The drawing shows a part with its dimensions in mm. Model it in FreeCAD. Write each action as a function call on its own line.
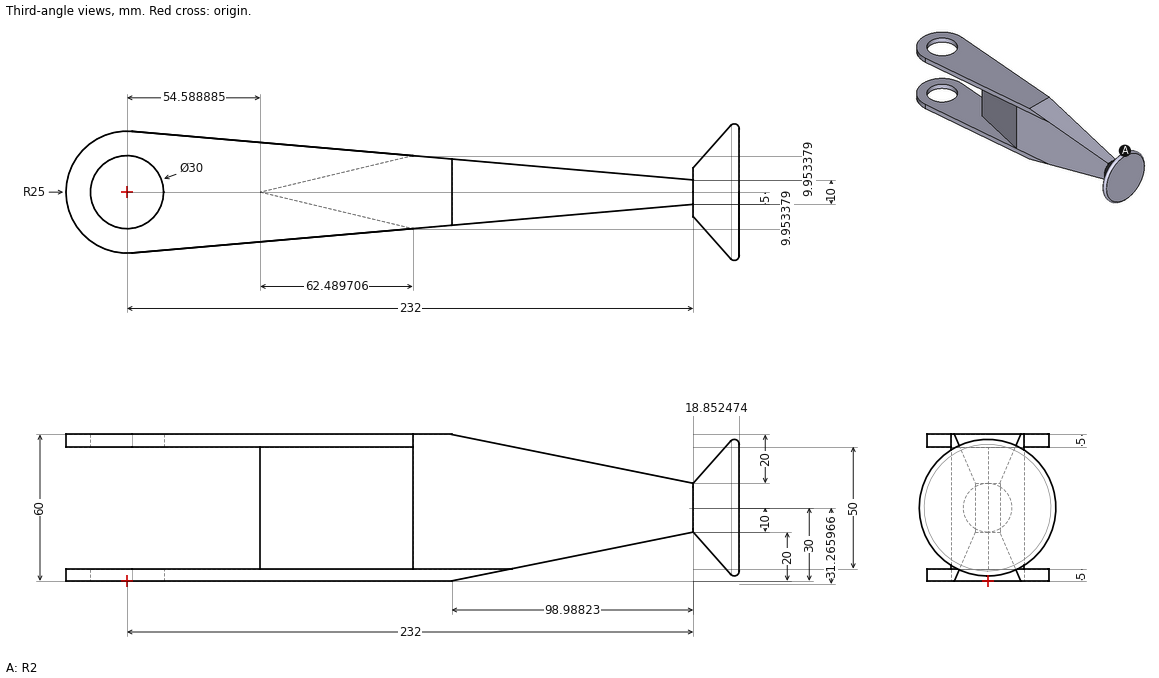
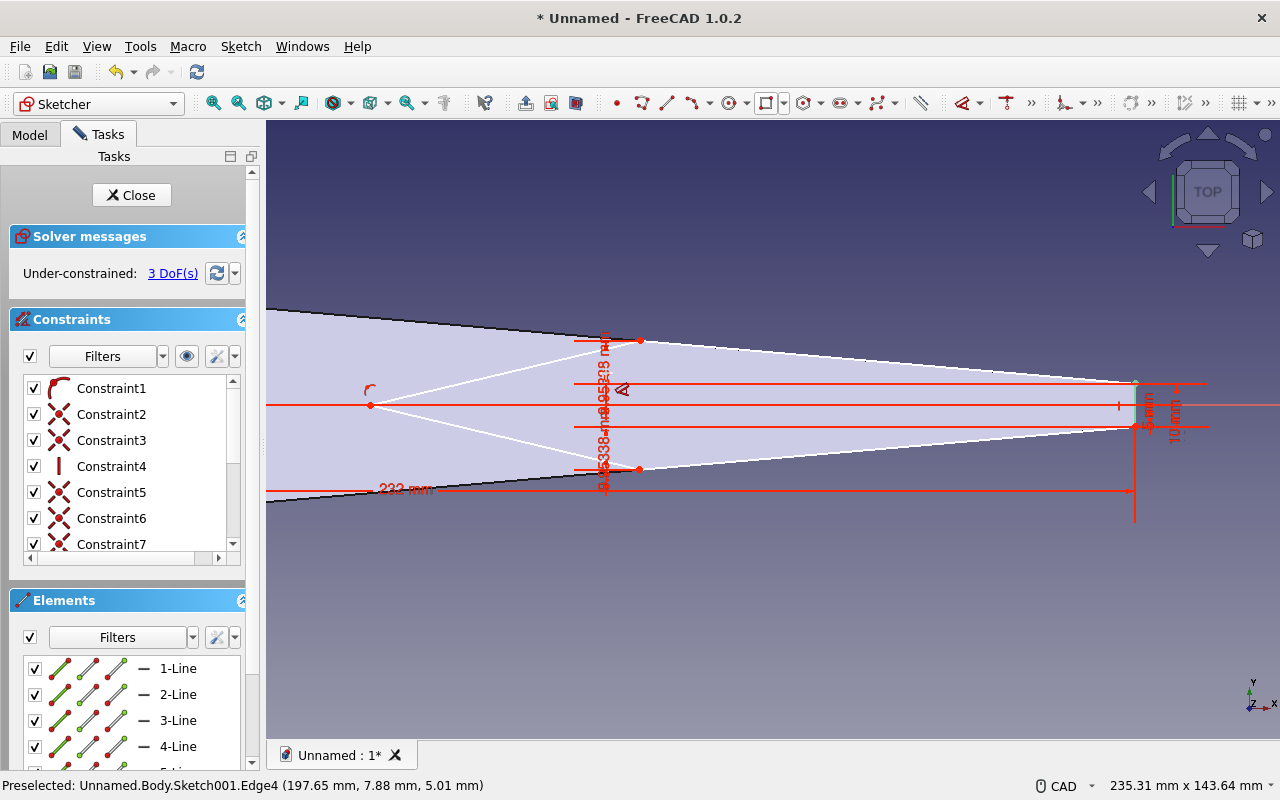
click(370, 405)
click(332, 439)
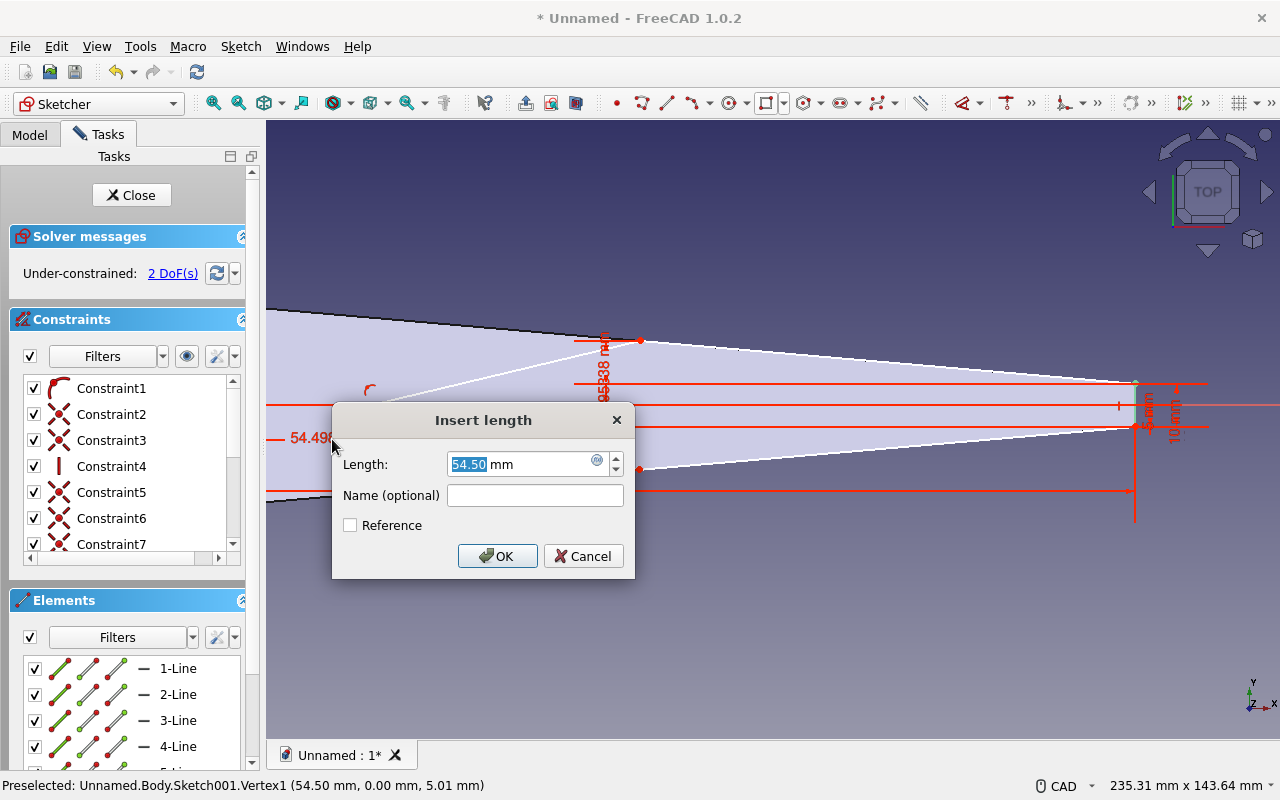
text(54.588885)
key(Return)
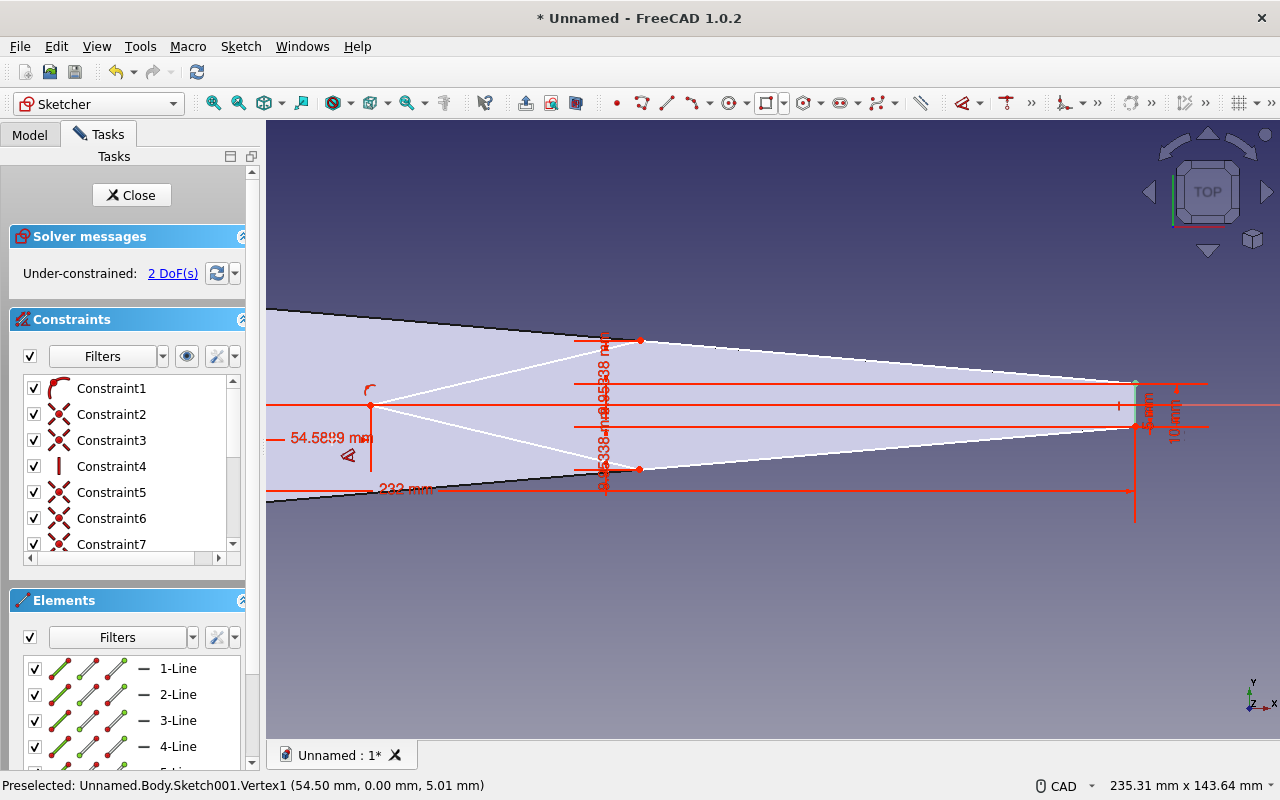
click(451, 425)
click(505, 504)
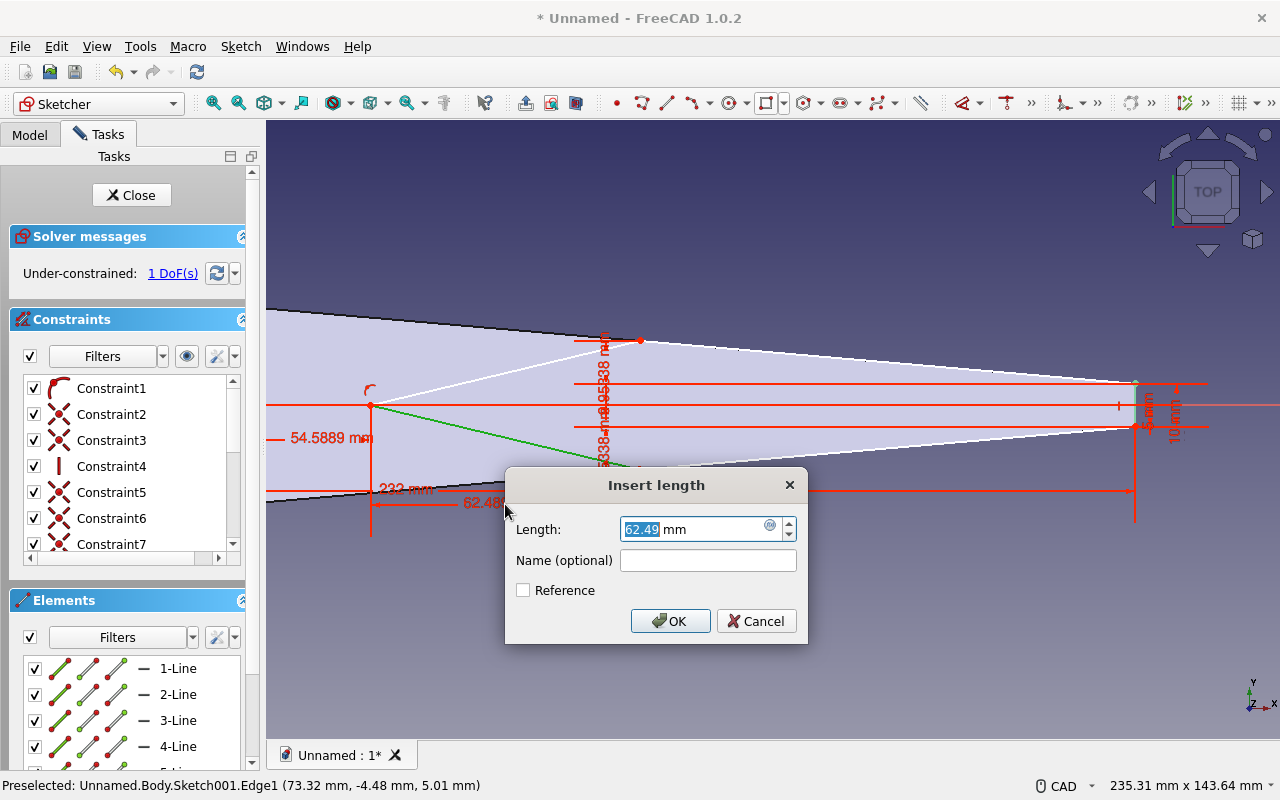
text(62.489706)
key(Return)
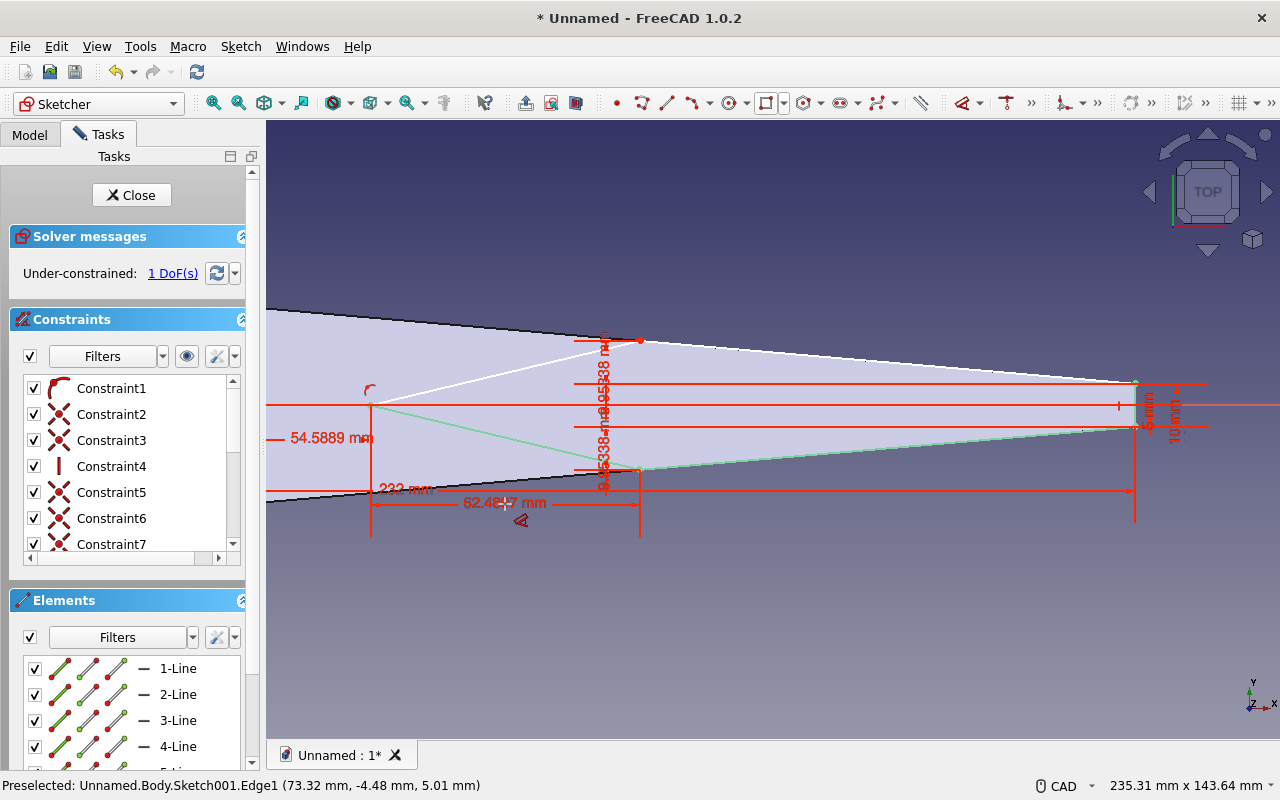
click(559, 360)
click(505, 307)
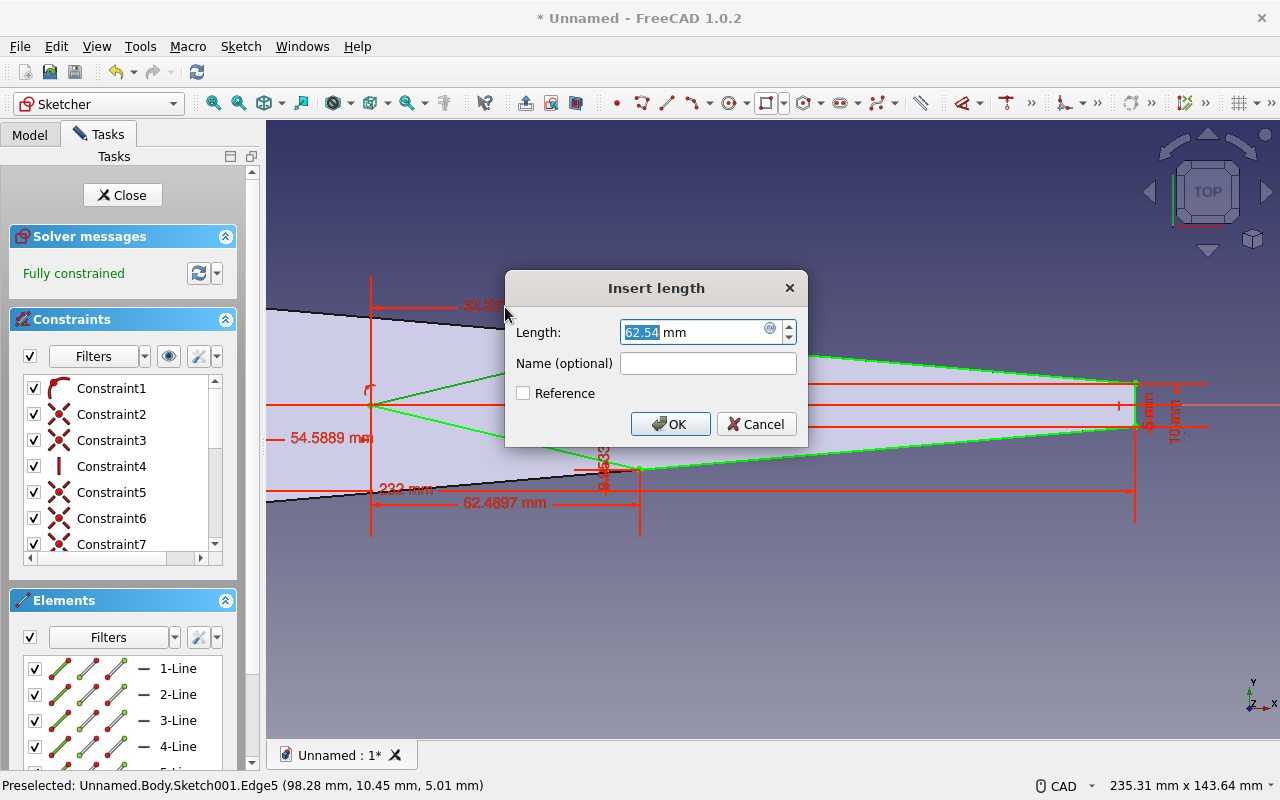
text(62.489706)
key(Return)
key(Escape)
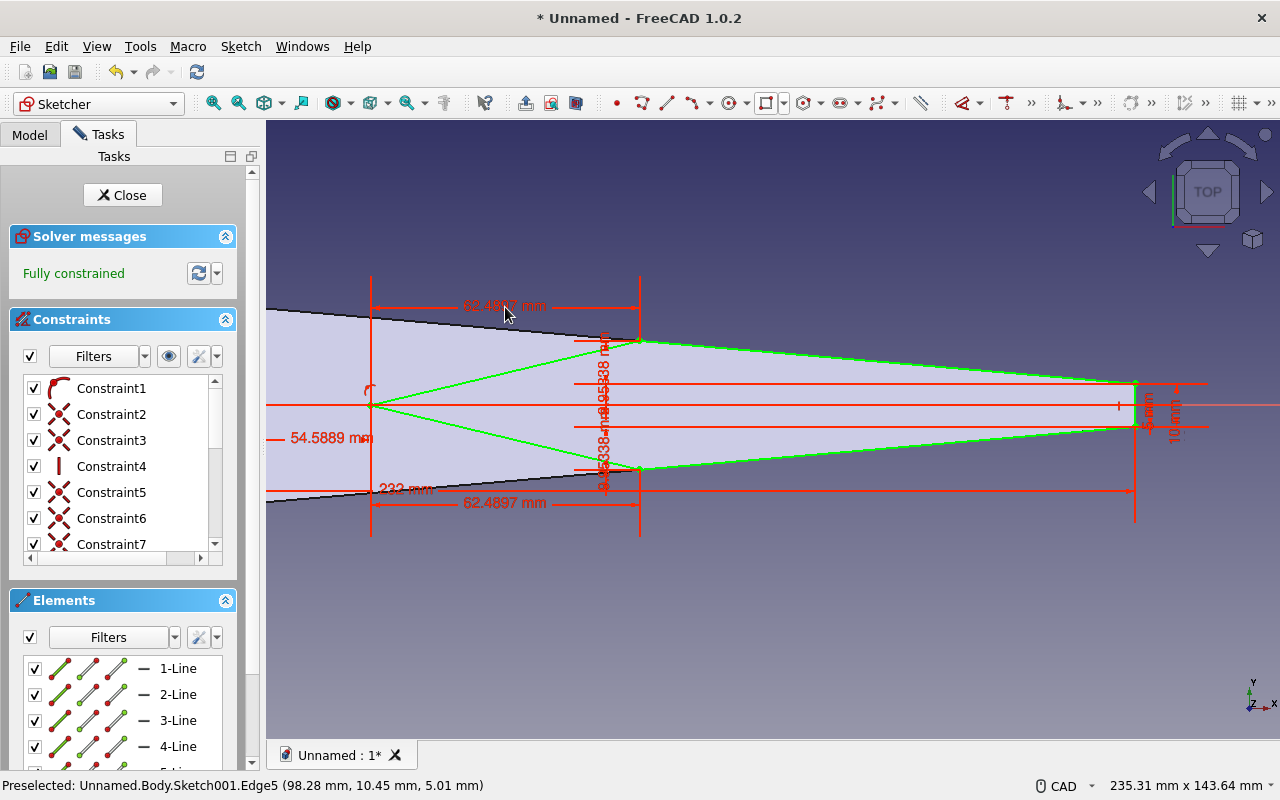
click(123, 195)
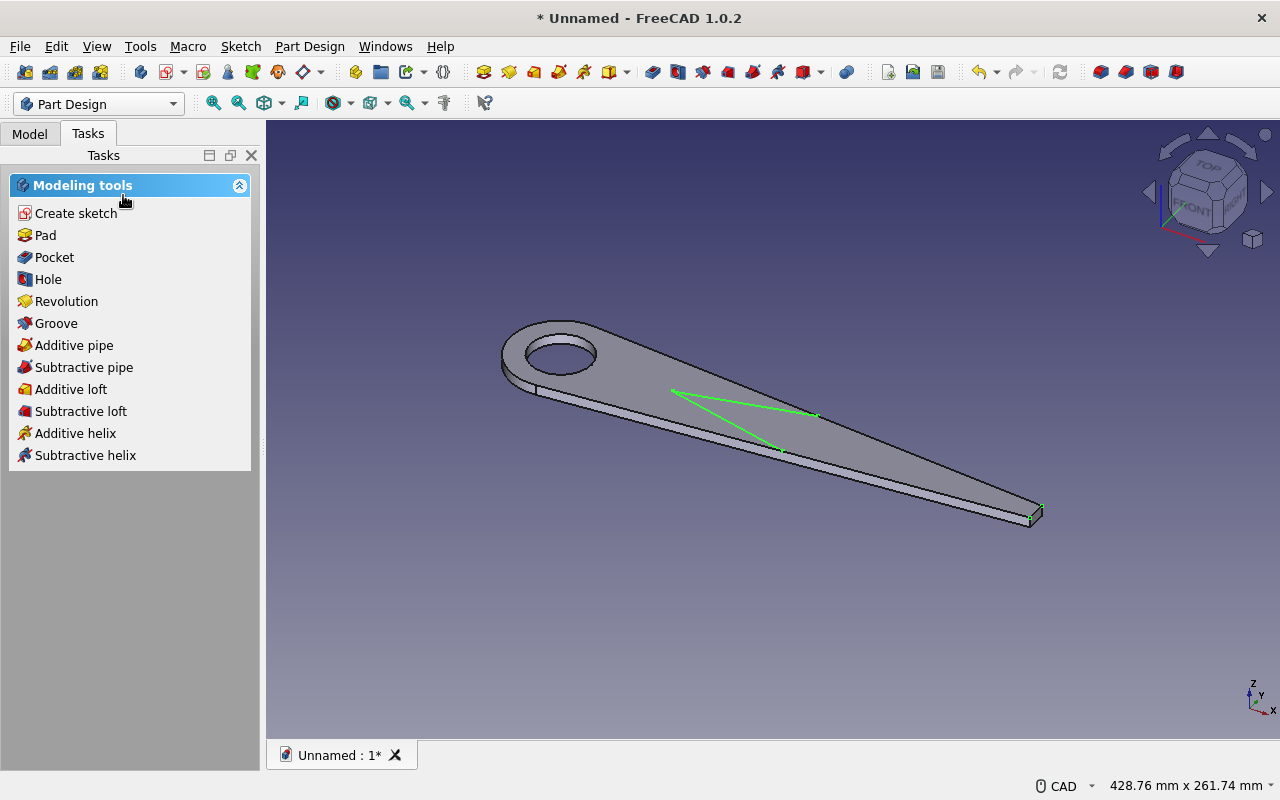
click(484, 72)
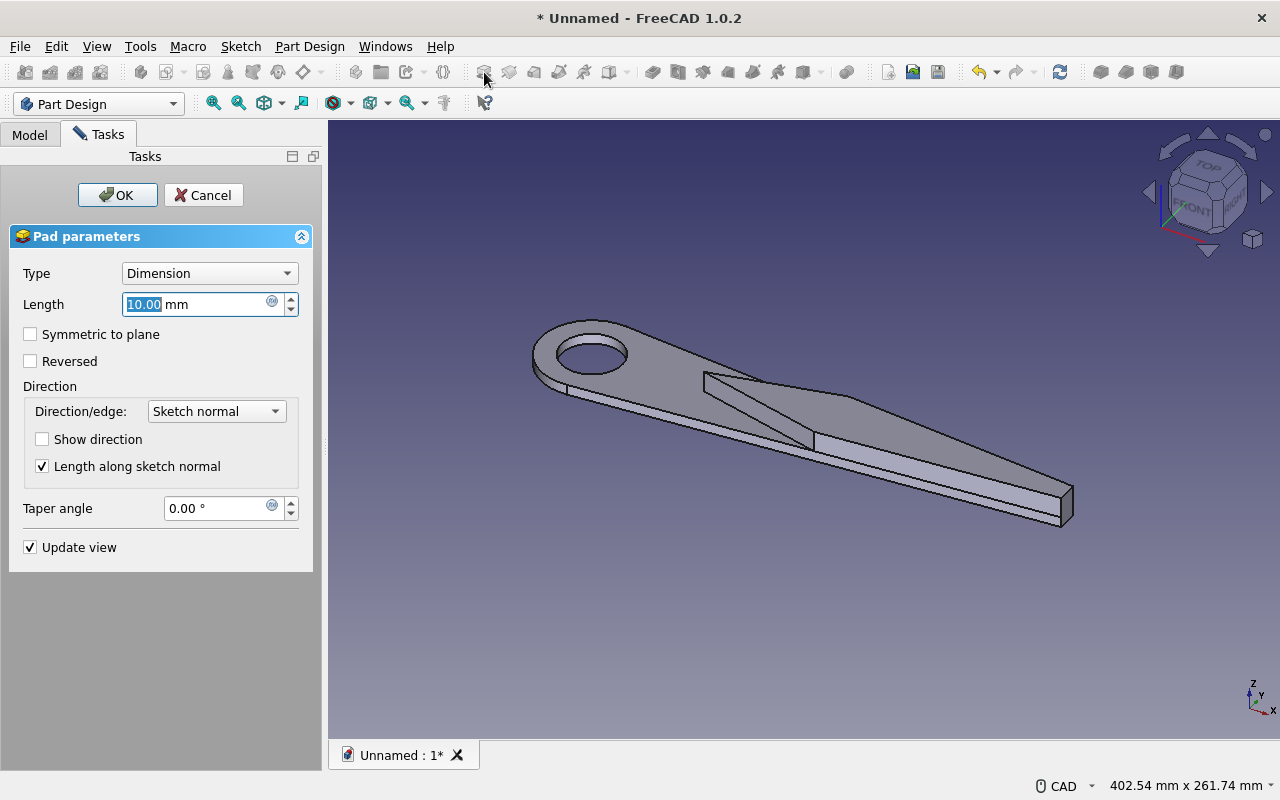
text(50)
key(Tab)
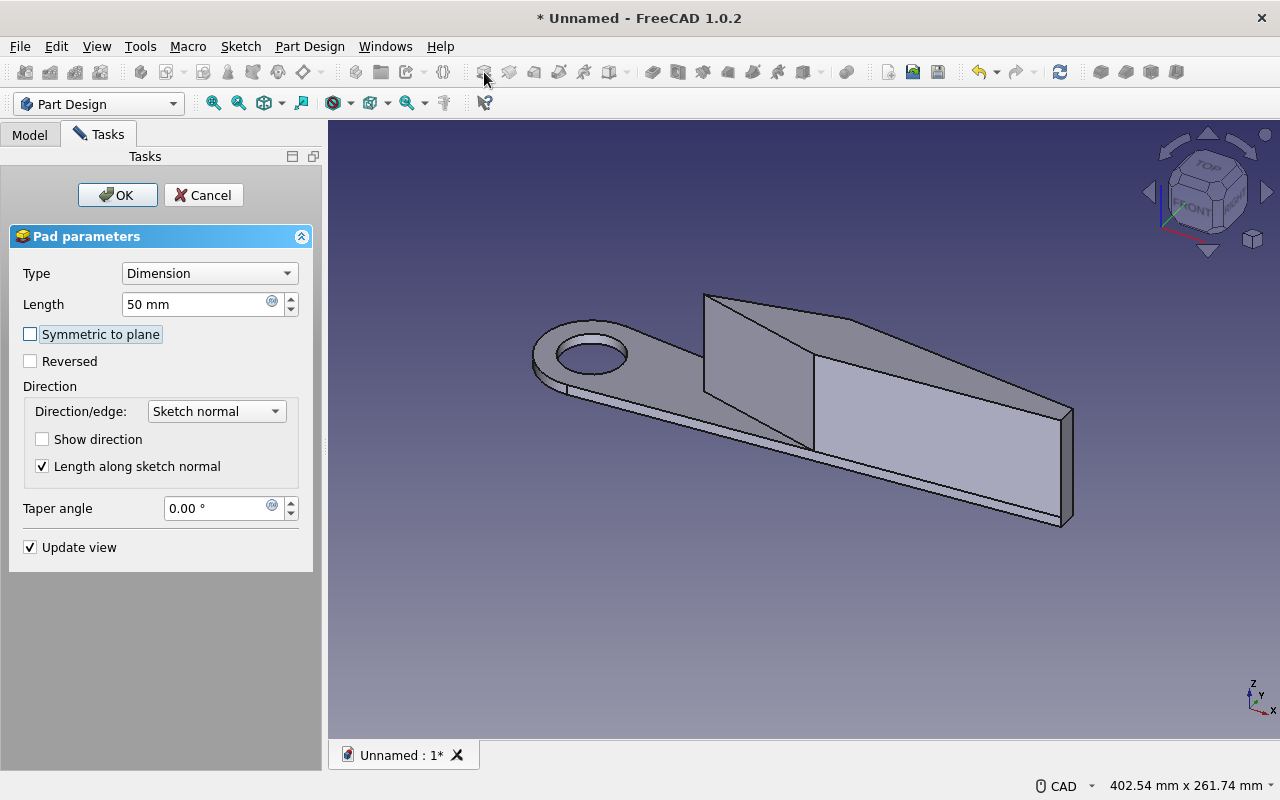
click(118, 195)